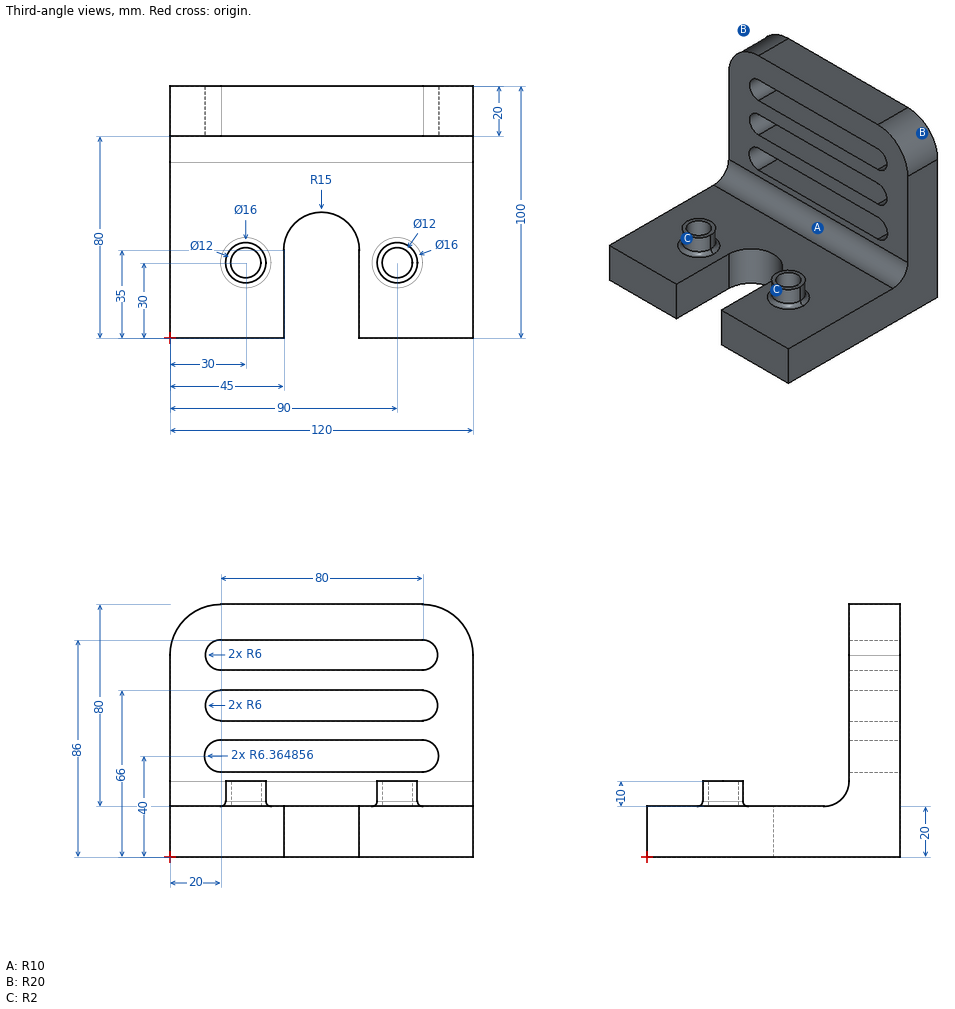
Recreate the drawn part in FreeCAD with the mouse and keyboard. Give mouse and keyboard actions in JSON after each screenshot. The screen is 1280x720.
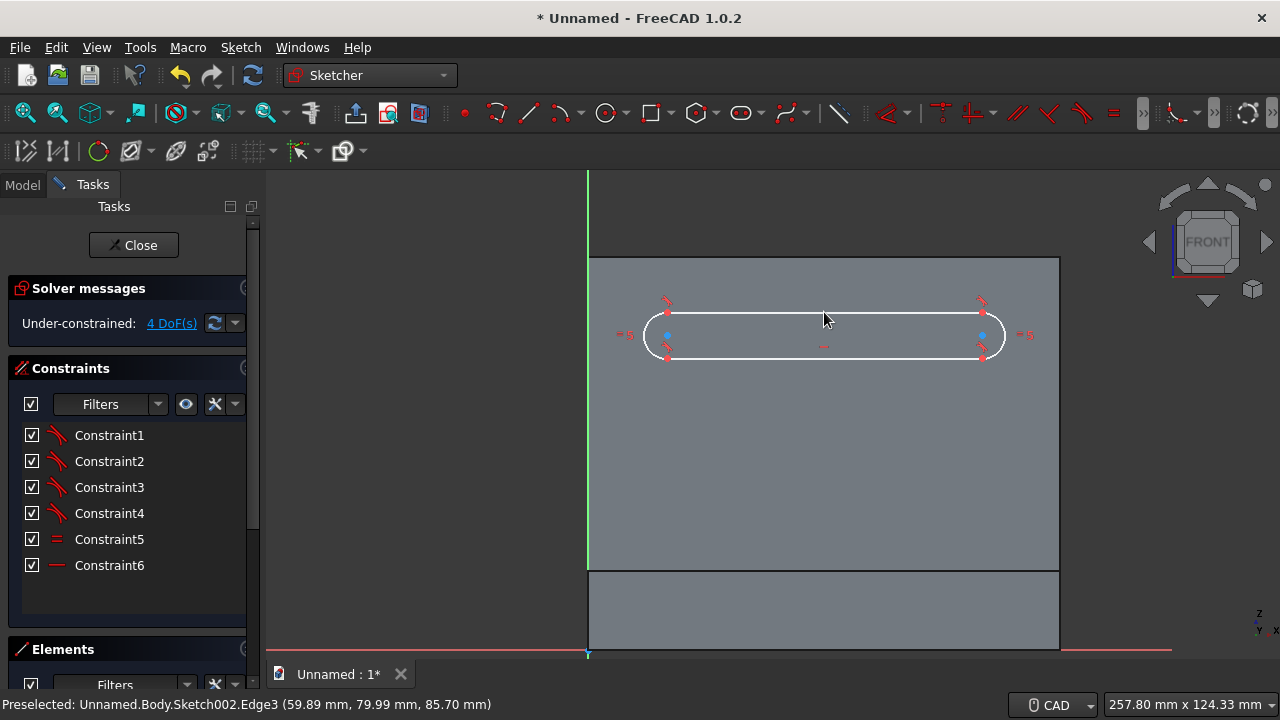
{"action": "left_click", "coordinate": [886, 114]}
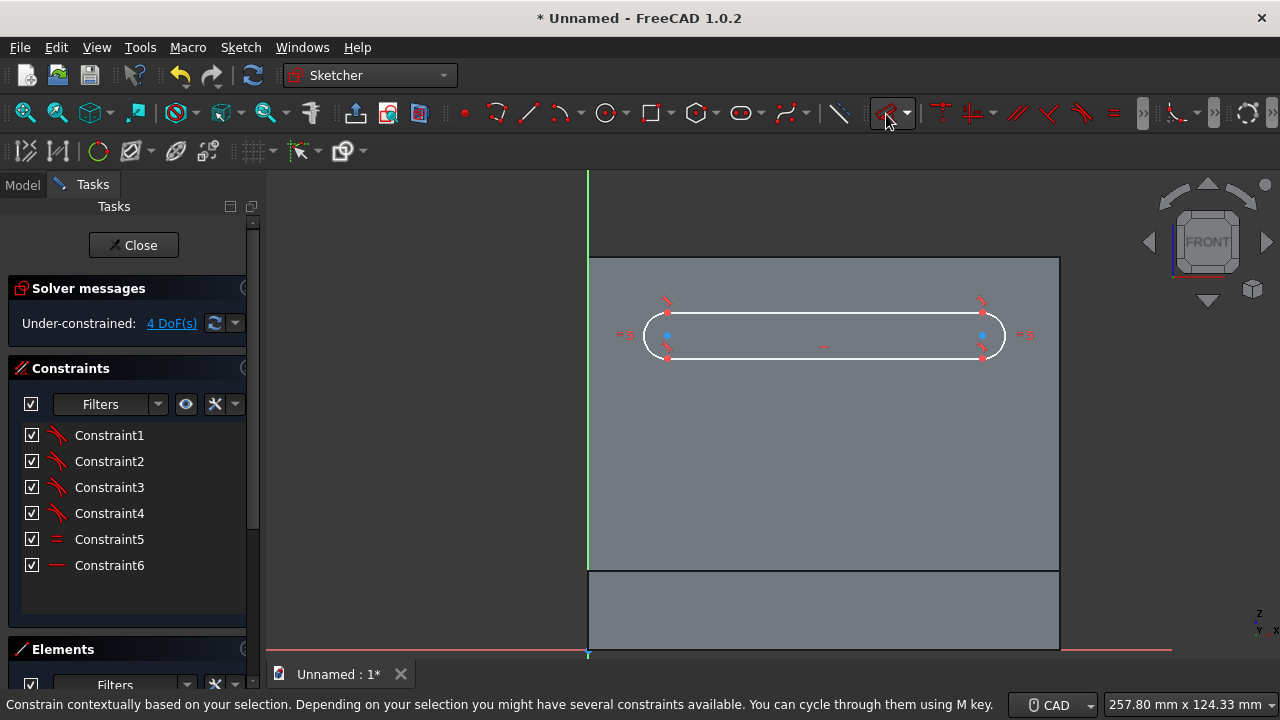
{"action": "scroll", "coordinate": [648, 322], "scroll_direction": "up", "scroll_amount": 3}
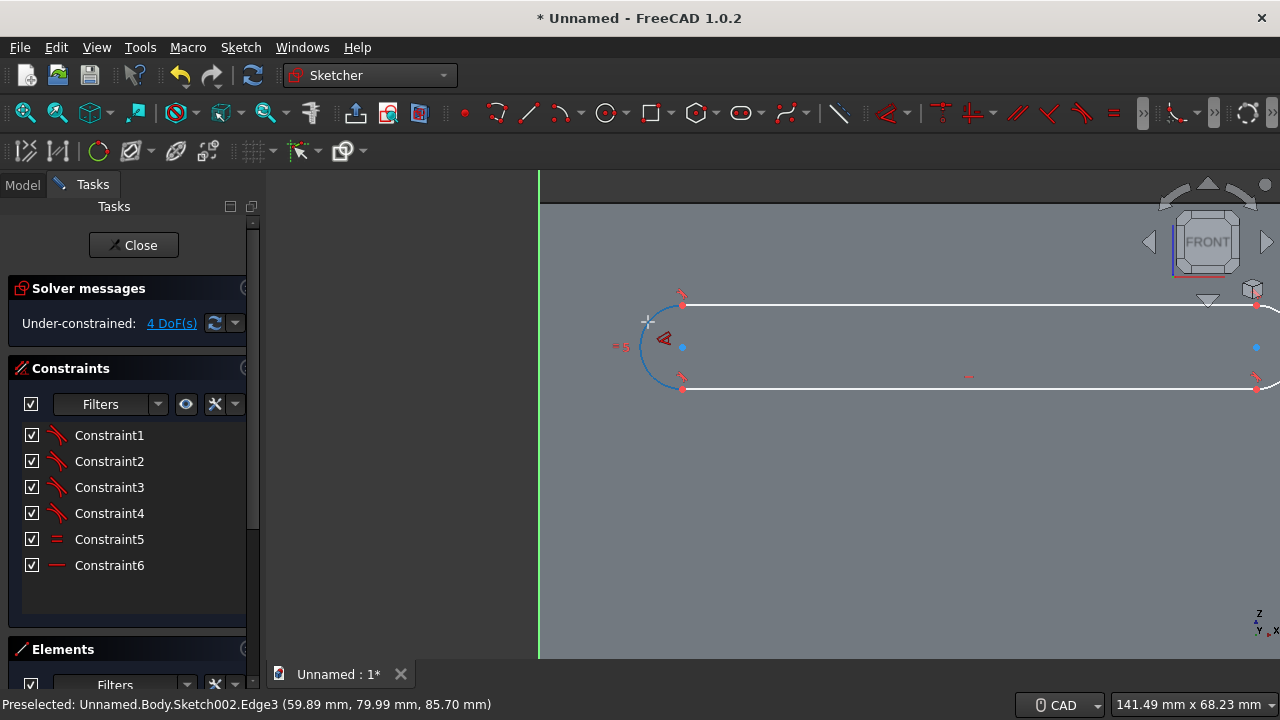
{"action": "left_click", "coordinate": [648, 323]}
{"action": "left_click", "coordinate": [622, 305]}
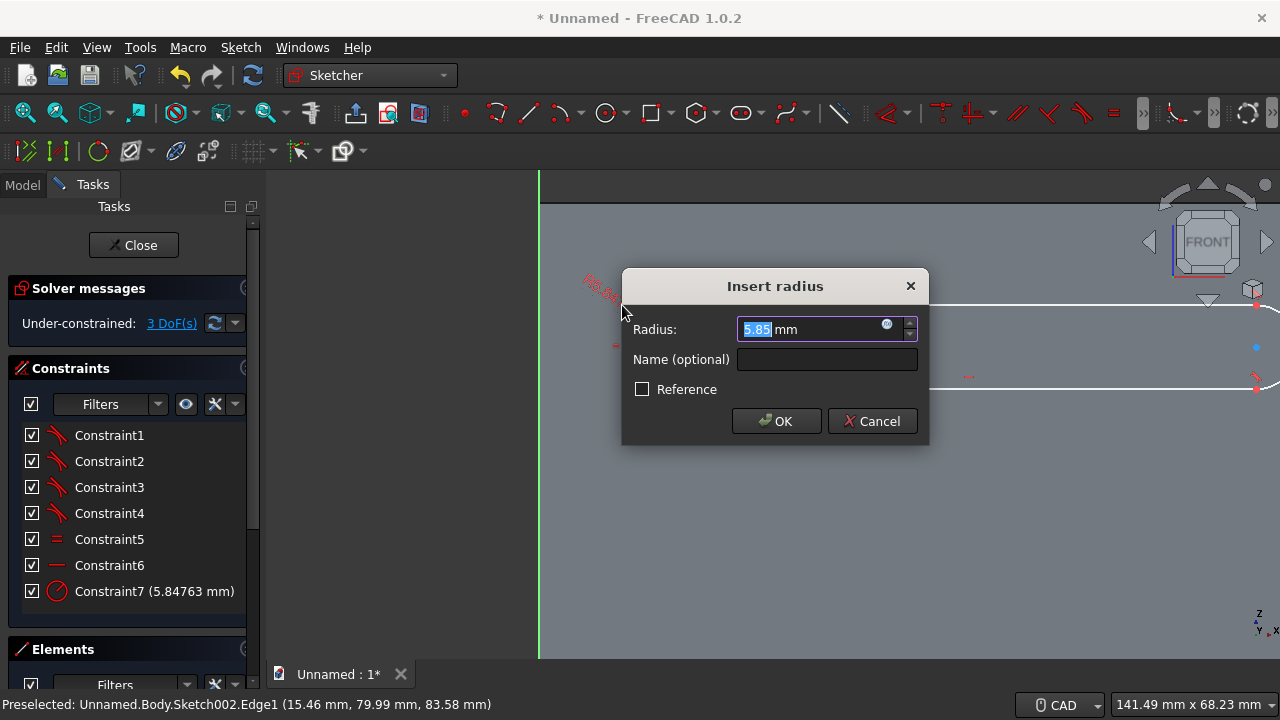
{"action": "type", "text": "6"}
{"action": "key", "text": "Return"}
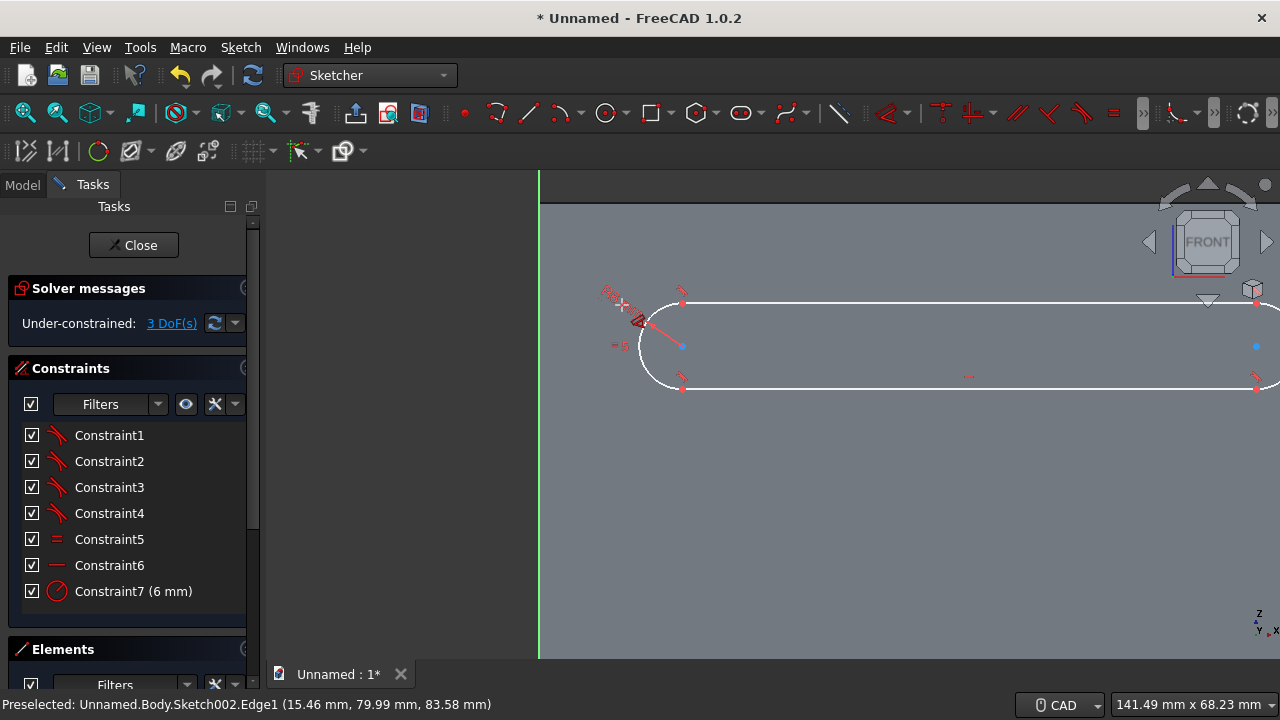
{"action": "left_click", "coordinate": [855, 303]}
{"action": "left_click", "coordinate": [899, 269]}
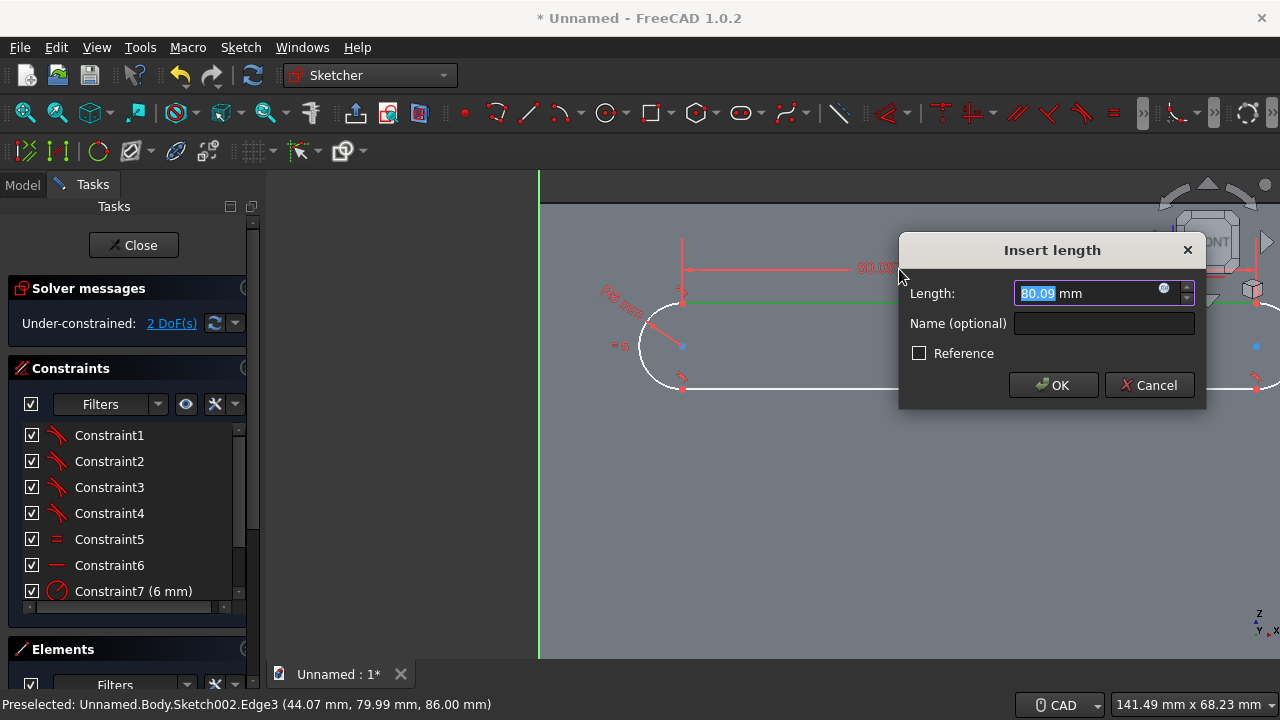
{"action": "type", "text": "80"}
{"action": "key", "text": "Return"}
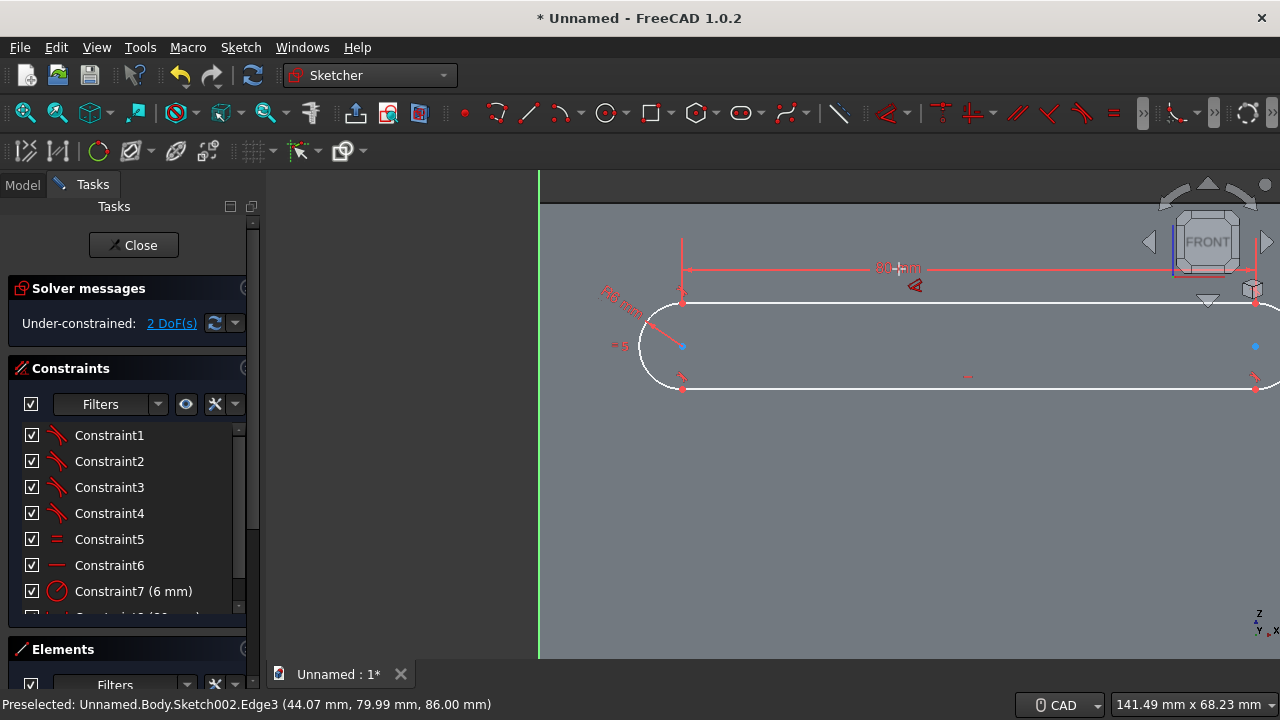
{"action": "left_click", "coordinate": [682, 303]}
{"action": "left_click", "coordinate": [611, 269]}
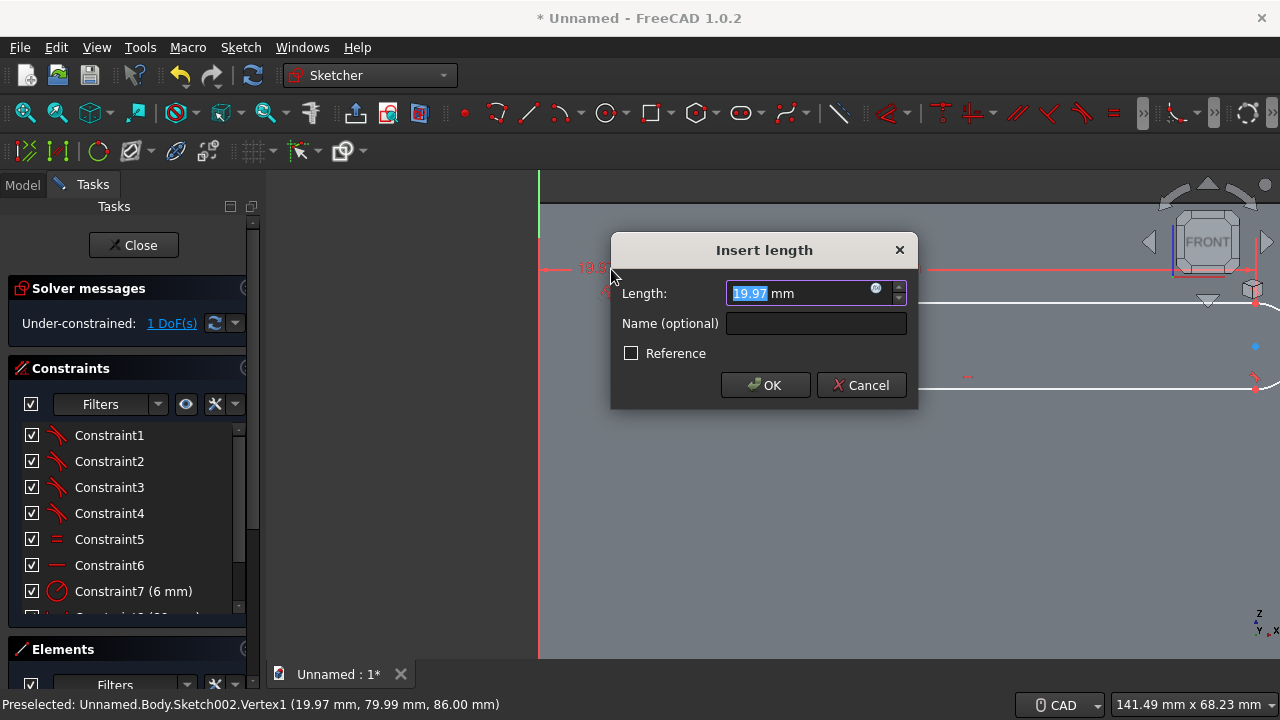
{"action": "type", "text": "20"}
{"action": "key", "text": "Return"}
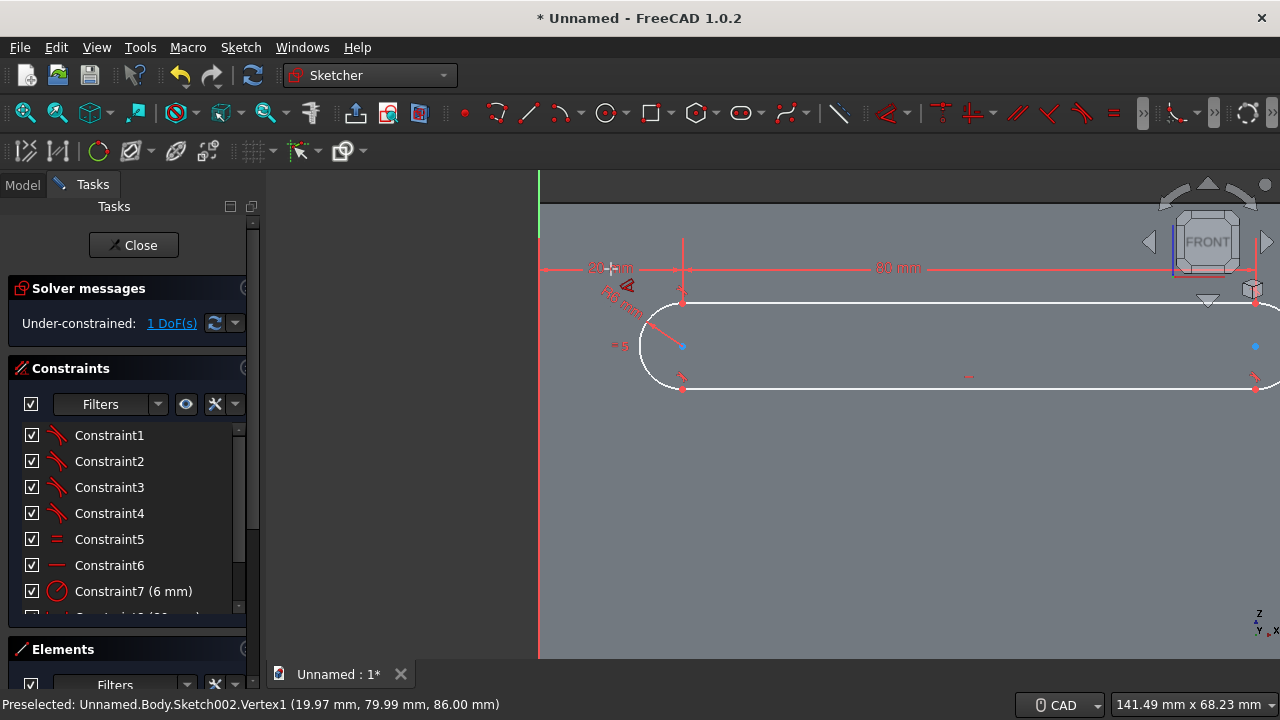
{"action": "left_click", "coordinate": [683, 303]}
{"action": "left_click", "coordinate": [505, 467]}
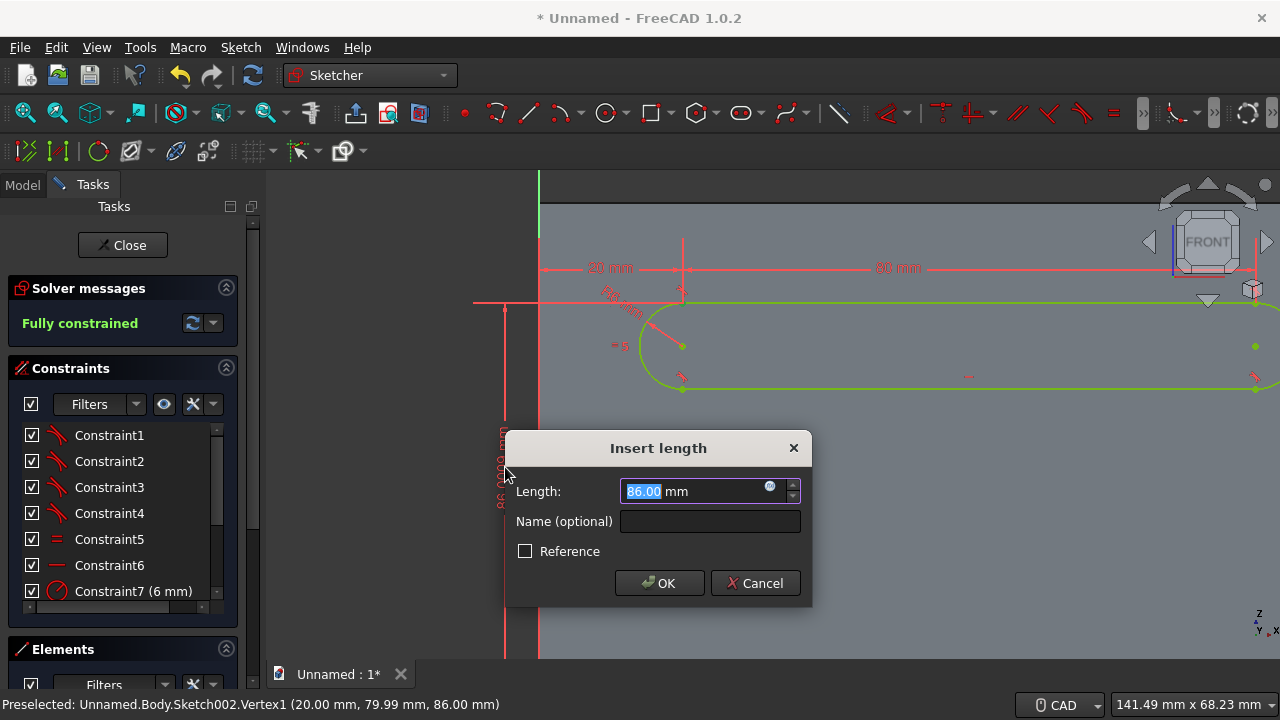
{"action": "type", "text": "86"}
{"action": "key", "text": "Return"}
{"action": "key", "text": "Escape"}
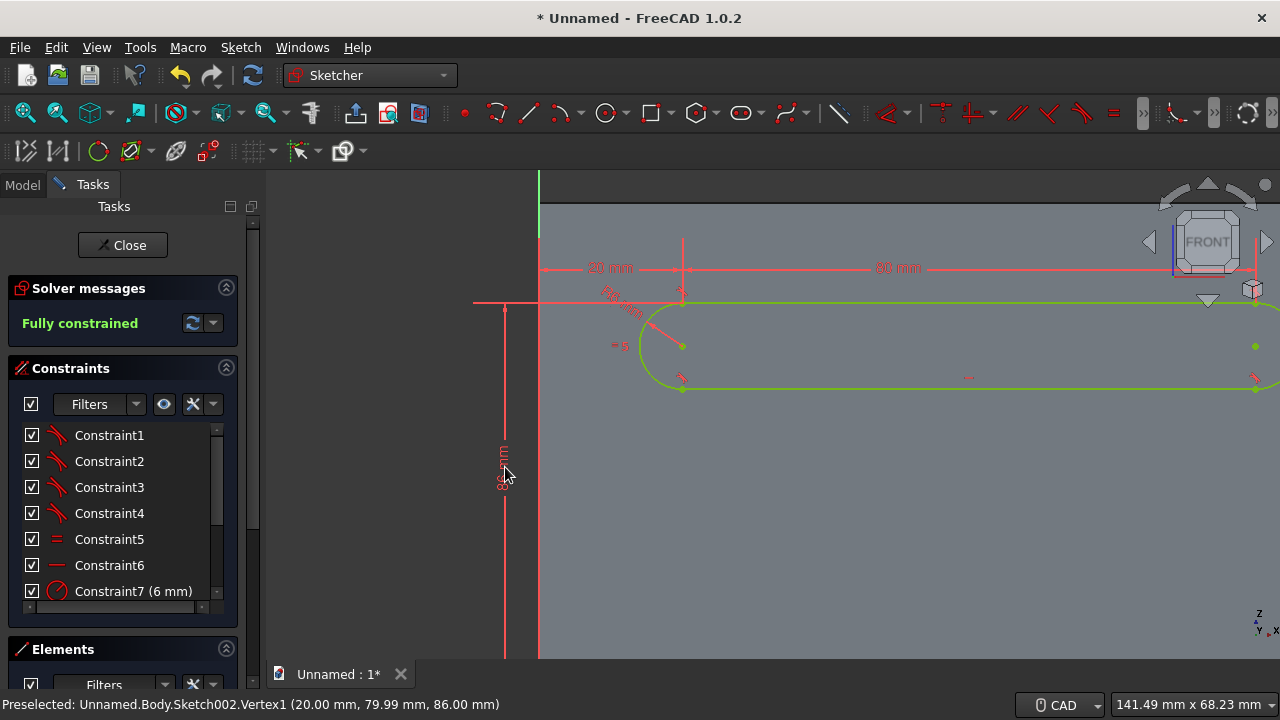
{"action": "left_click", "coordinate": [123, 245]}